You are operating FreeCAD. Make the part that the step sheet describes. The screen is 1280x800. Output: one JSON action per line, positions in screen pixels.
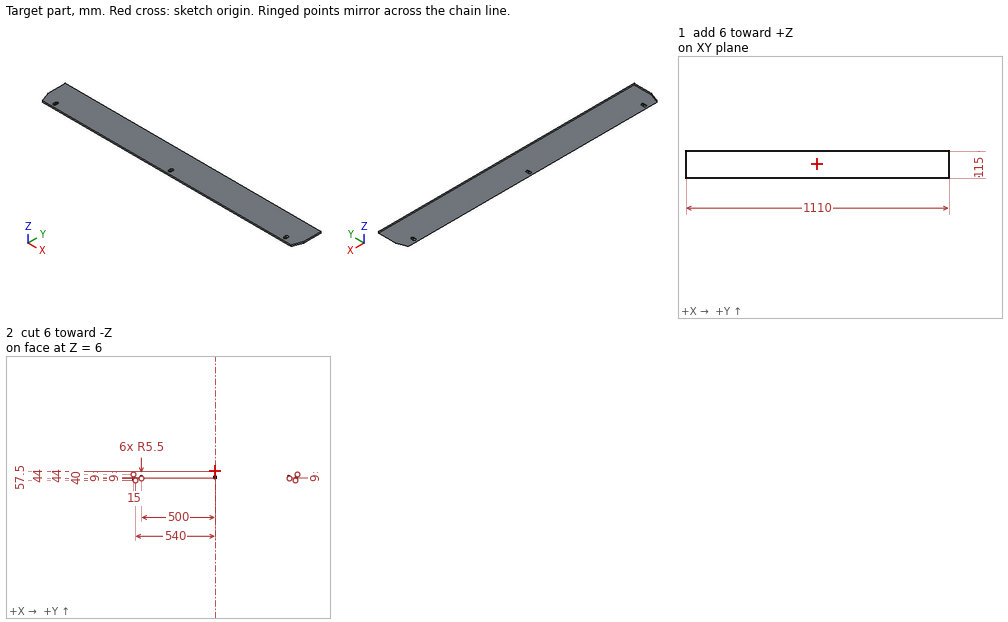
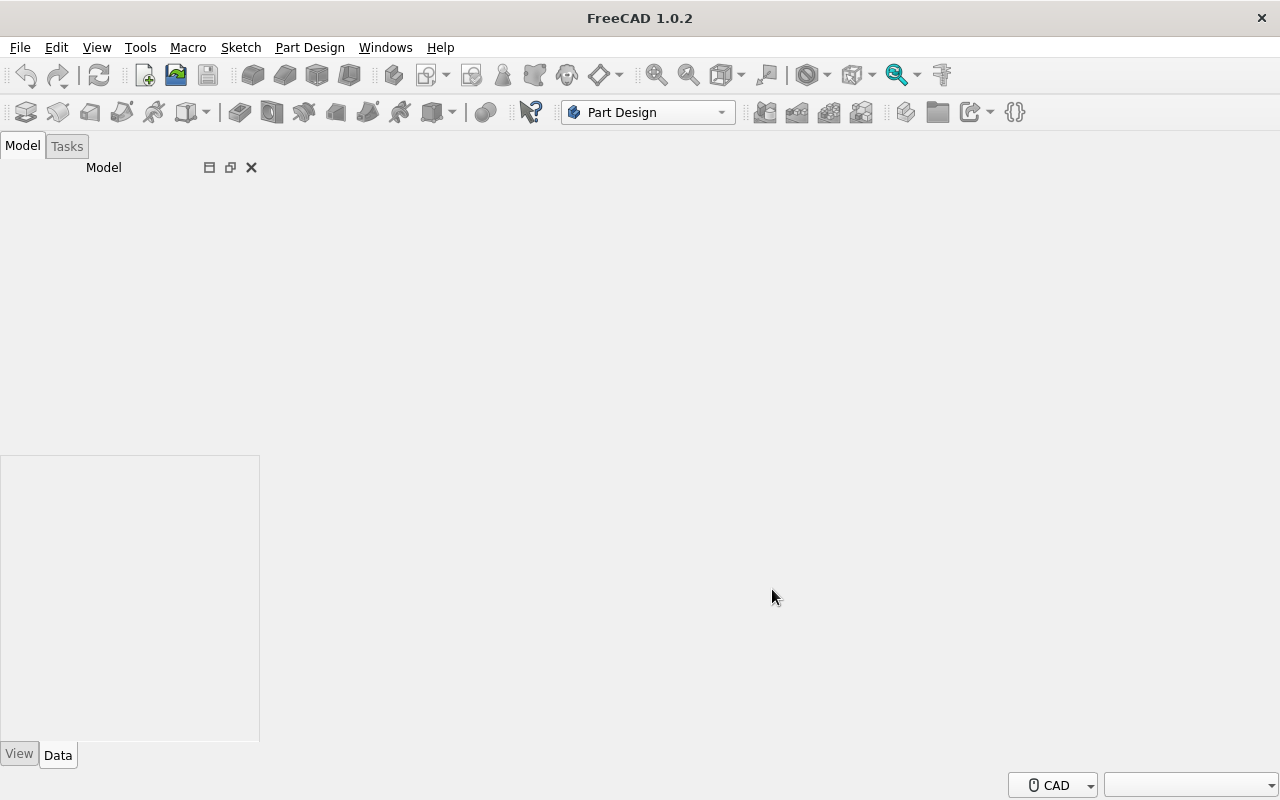
{"action": "left_click", "coordinate": [144, 76]}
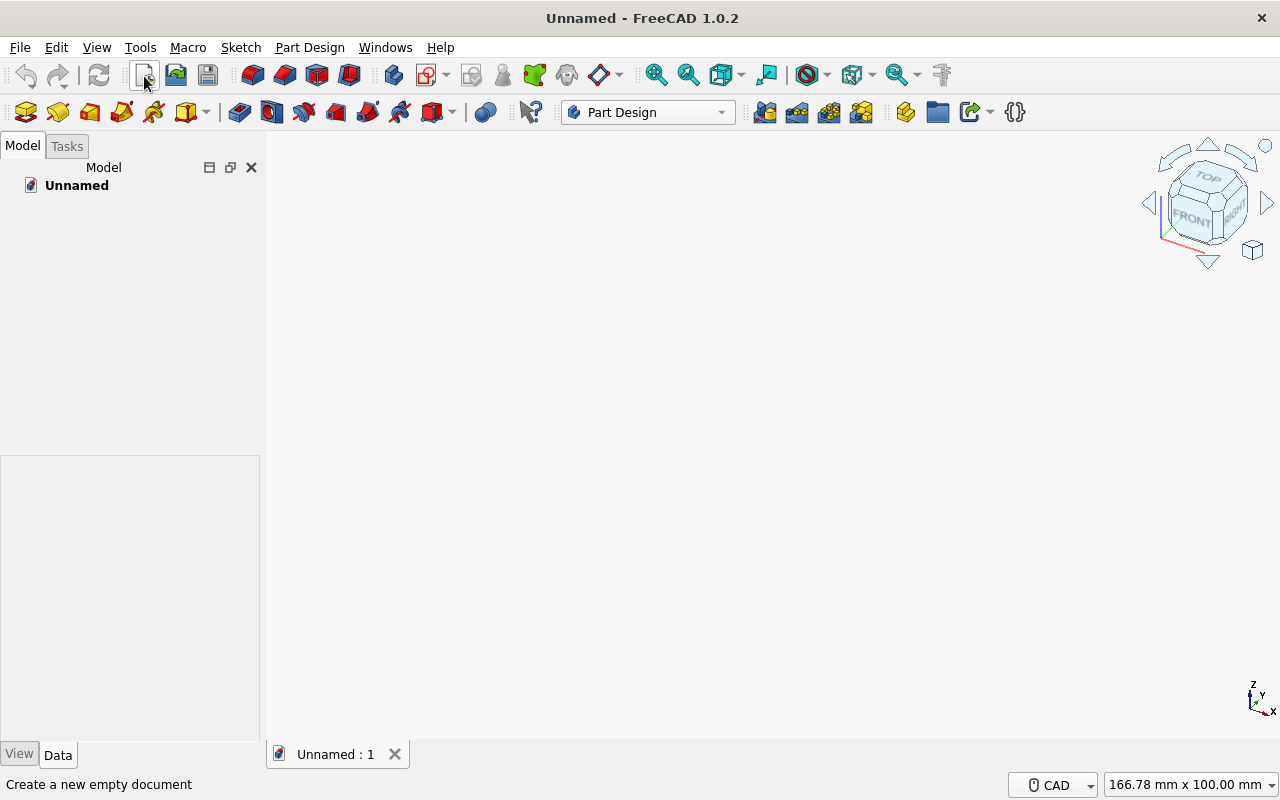
{"action": "left_click", "coordinate": [426, 76]}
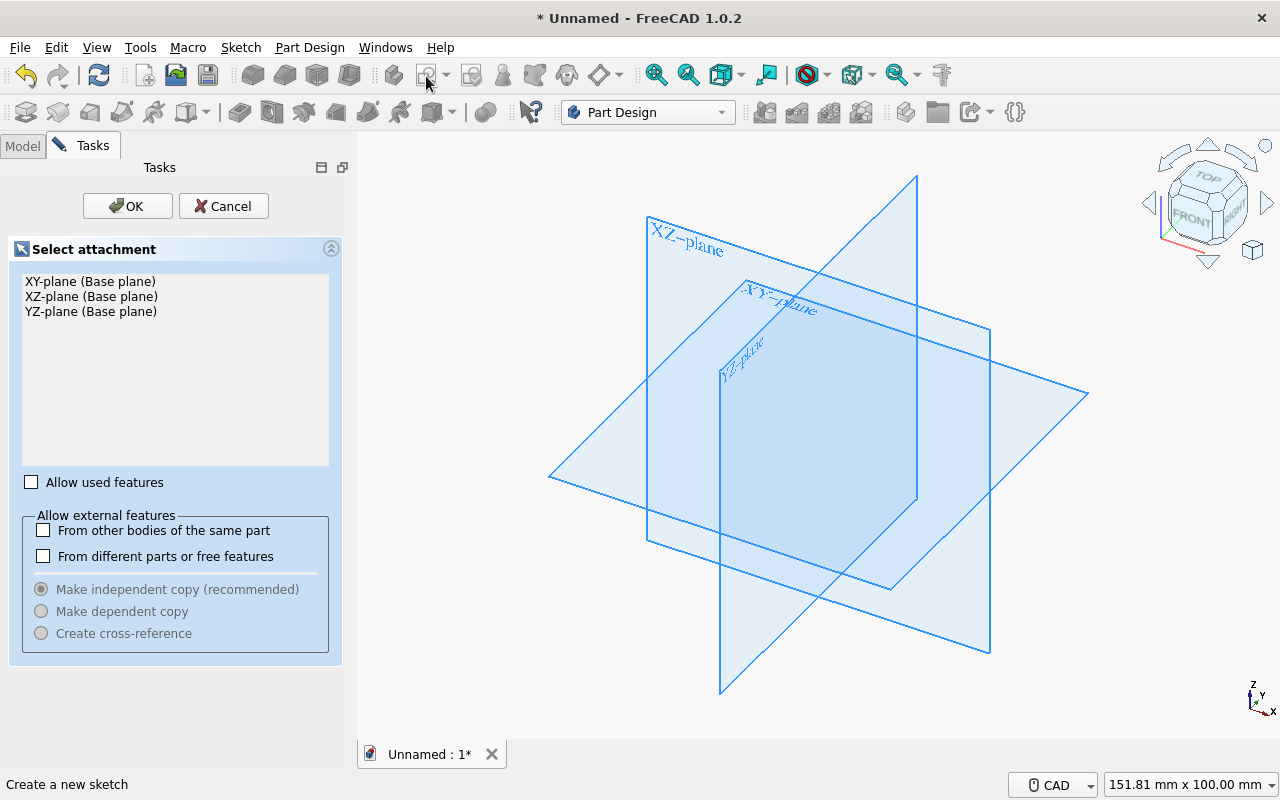
{"action": "left_click", "coordinate": [82, 282]}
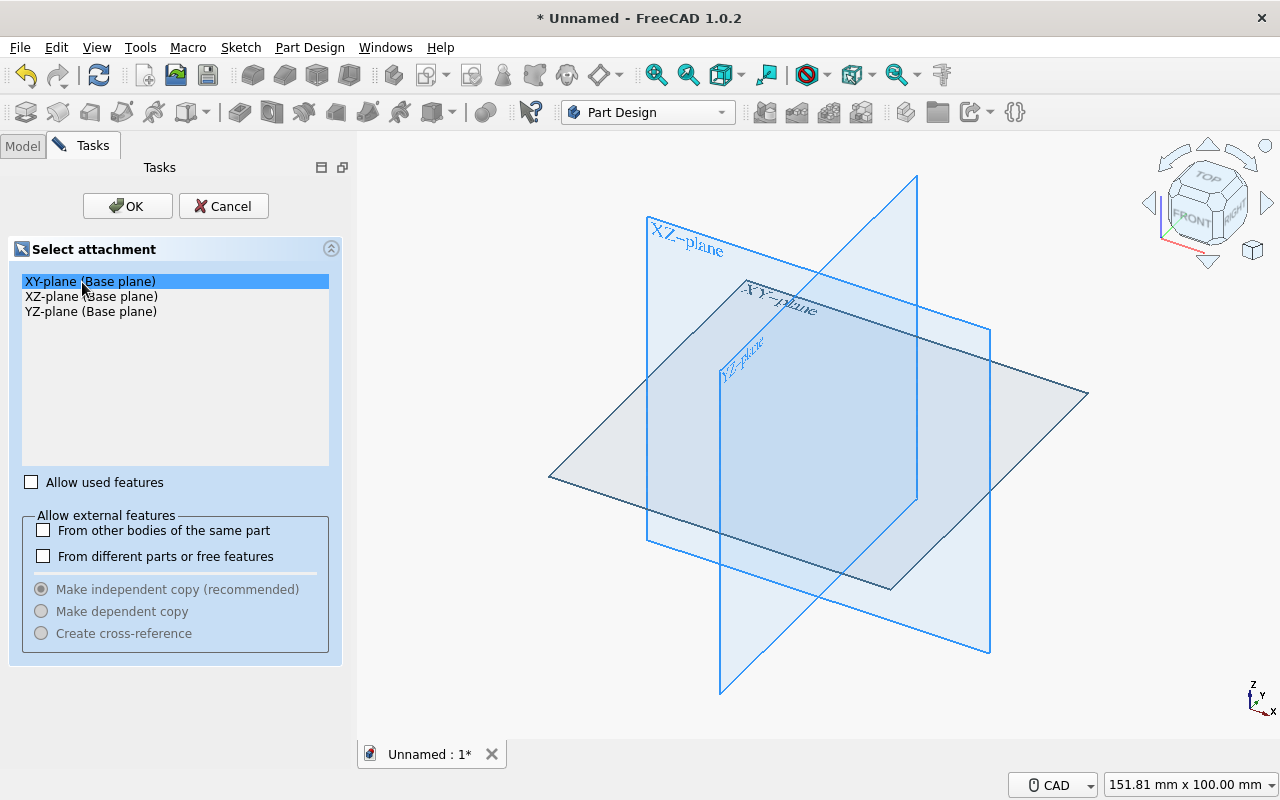
{"action": "left_click", "coordinate": [128, 206]}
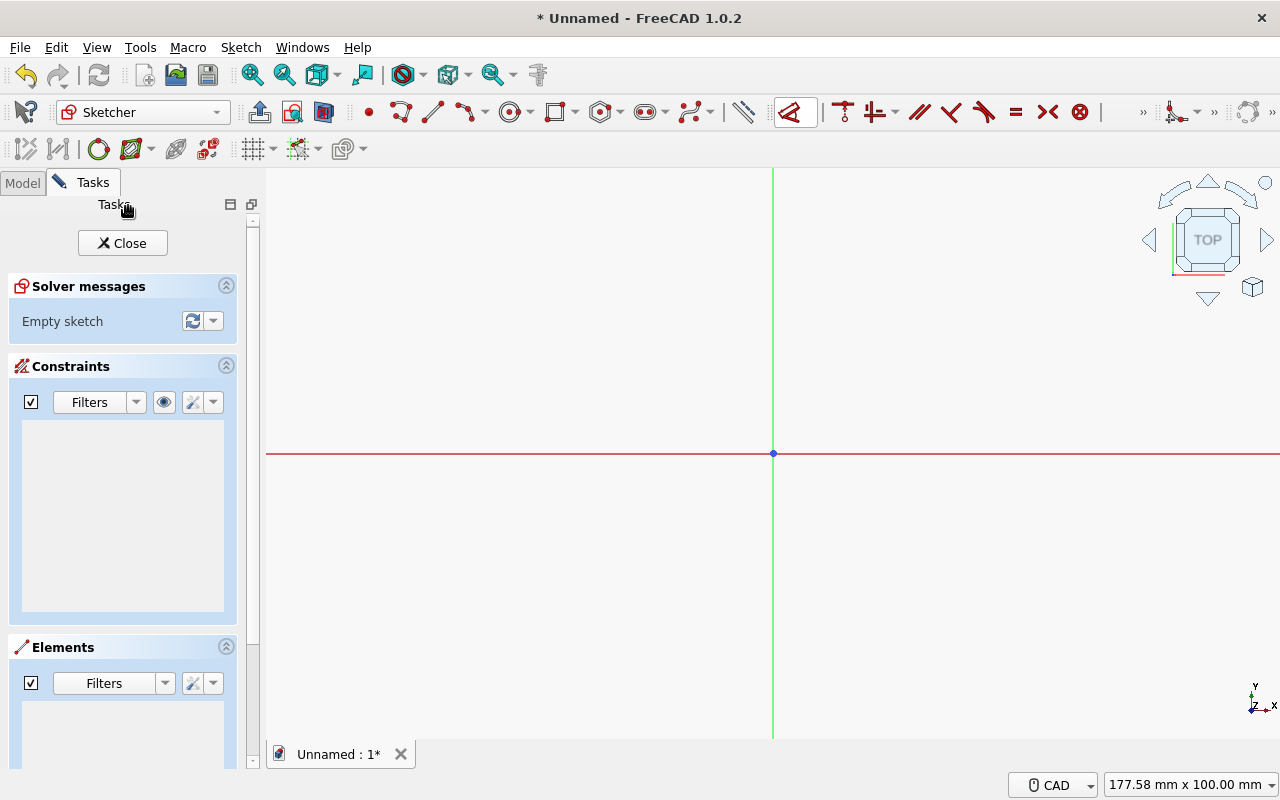
{"action": "scroll", "coordinate": [698, 454], "scroll_direction": "down", "scroll_amount": 12}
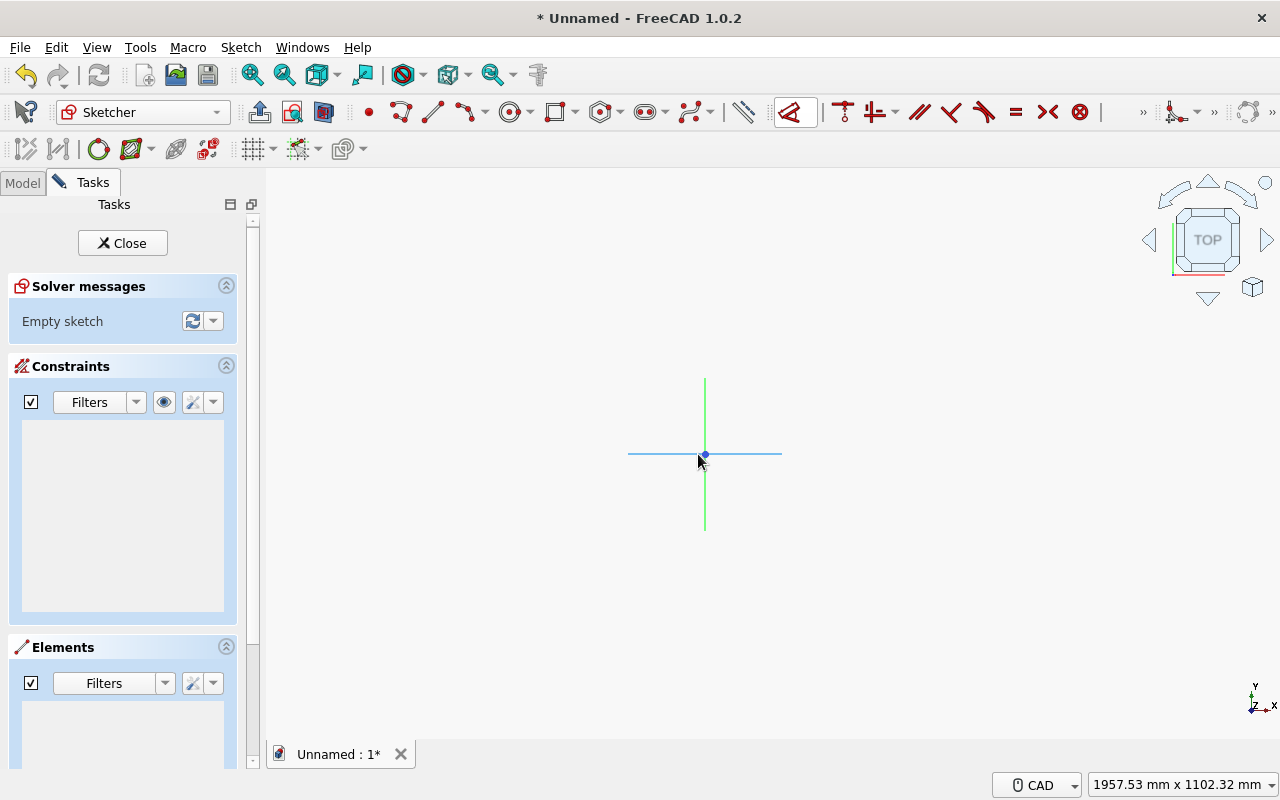
{"action": "key", "text": "g v"}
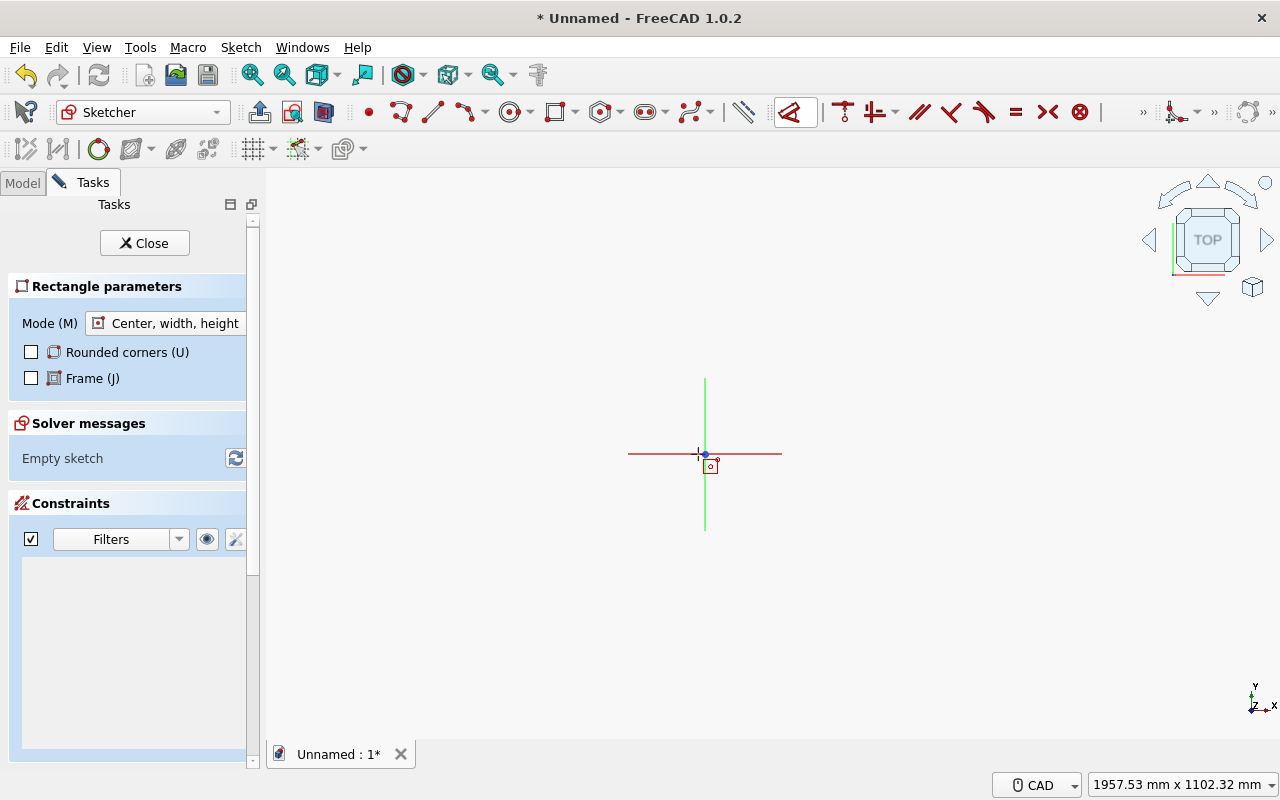
{"action": "left_click", "coordinate": [705, 454]}
{"action": "mouse_move", "coordinate": [993, 425]}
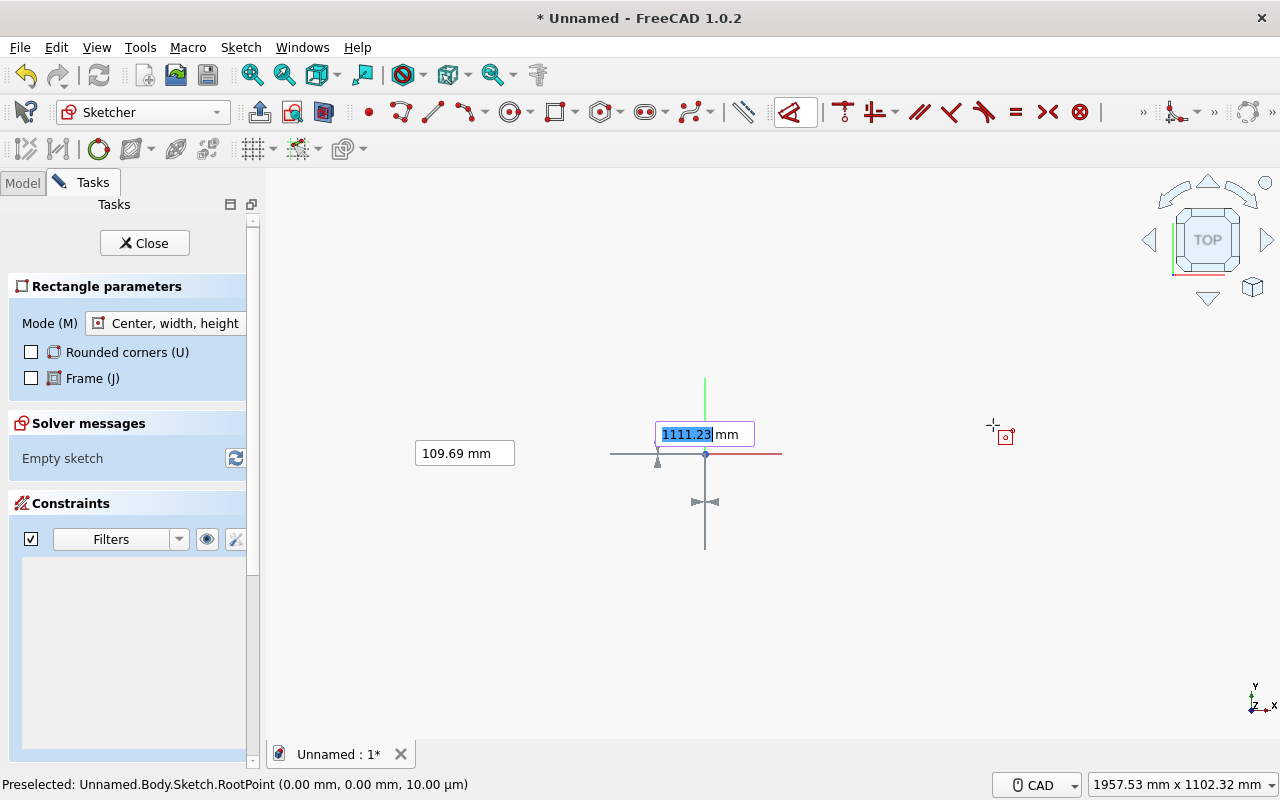
{"action": "type", "text": "1110"}
{"action": "key", "text": "Tab"}
{"action": "type", "text": "115"}
{"action": "key", "text": "Return"}
{"action": "key", "text": "Escape"}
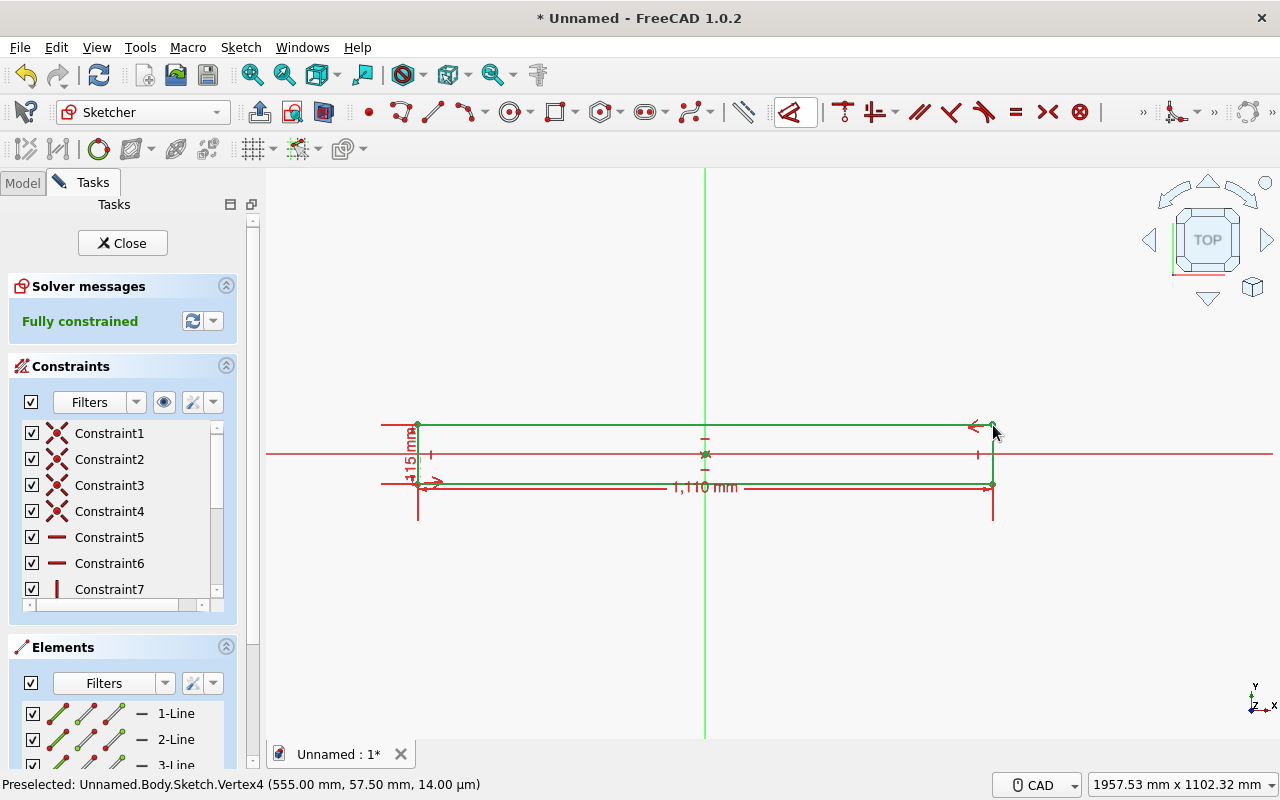
{"action": "left_click", "coordinate": [123, 243]}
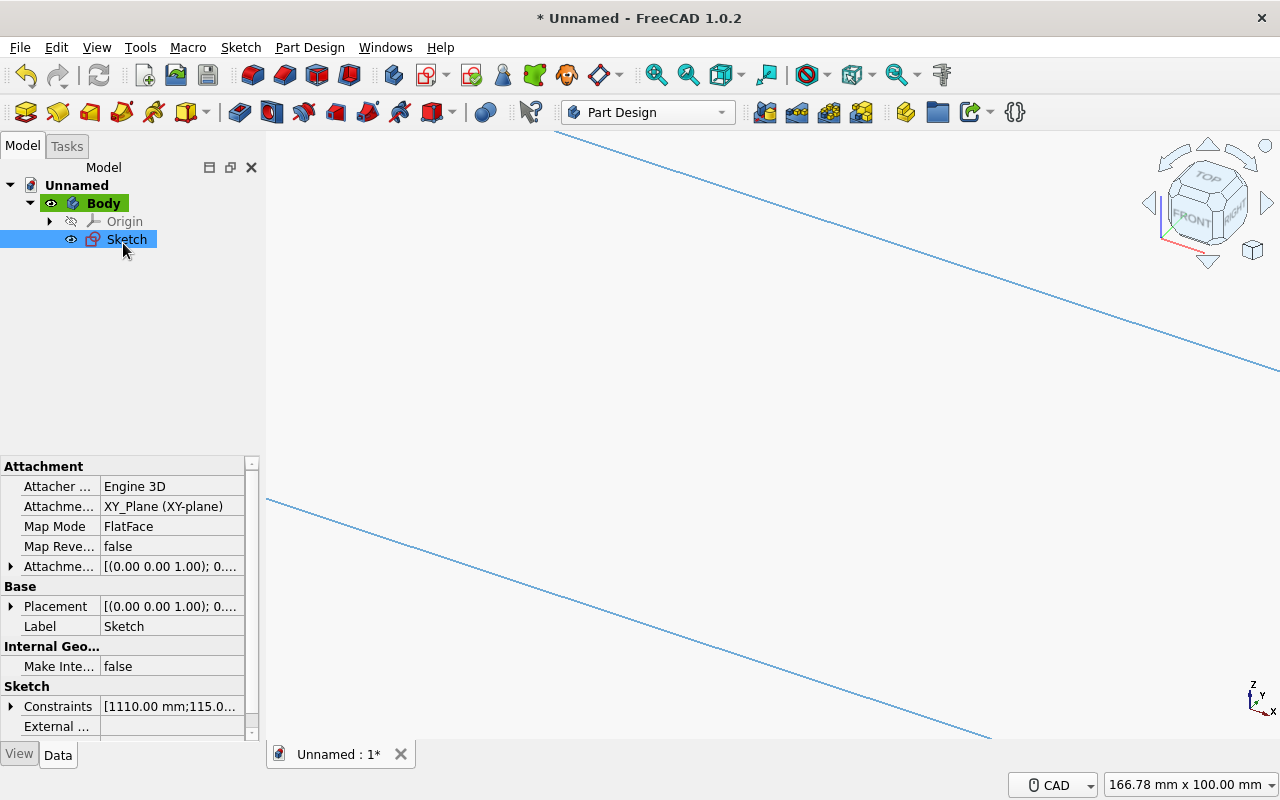
{"action": "left_click", "coordinate": [26, 112]}